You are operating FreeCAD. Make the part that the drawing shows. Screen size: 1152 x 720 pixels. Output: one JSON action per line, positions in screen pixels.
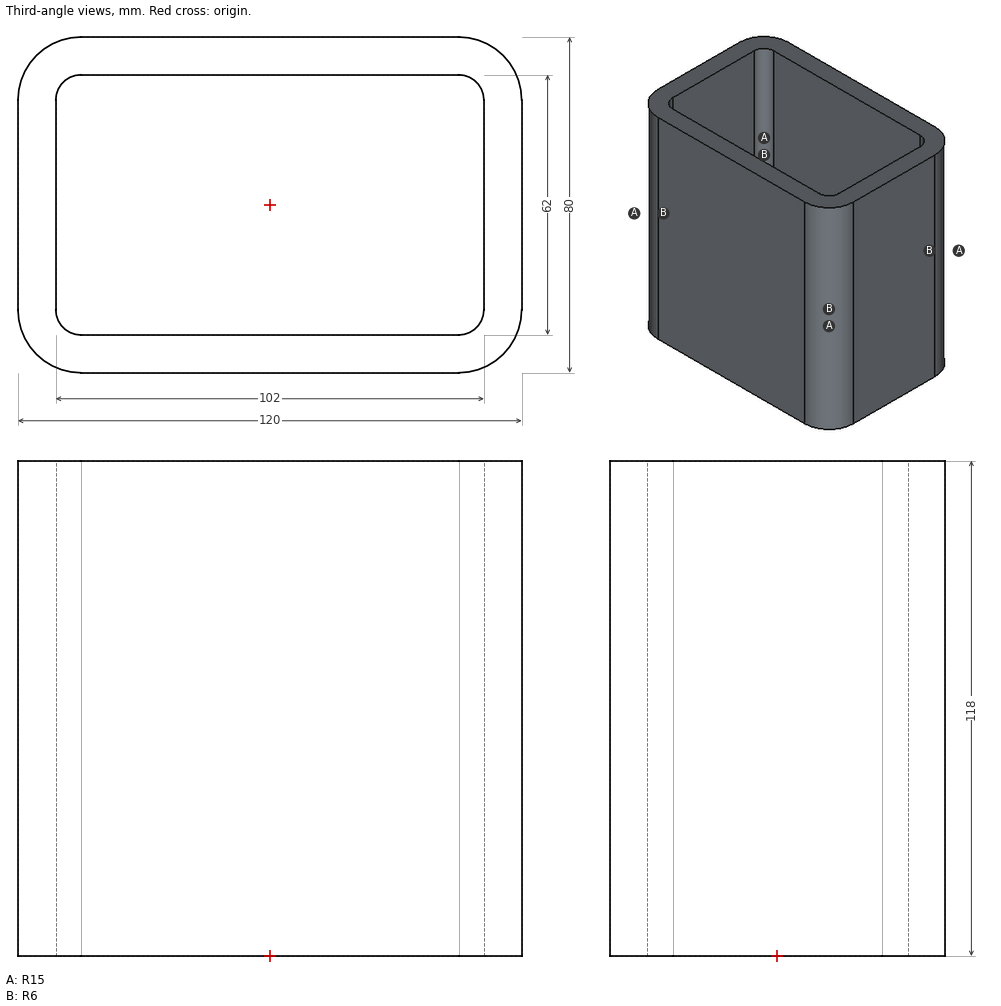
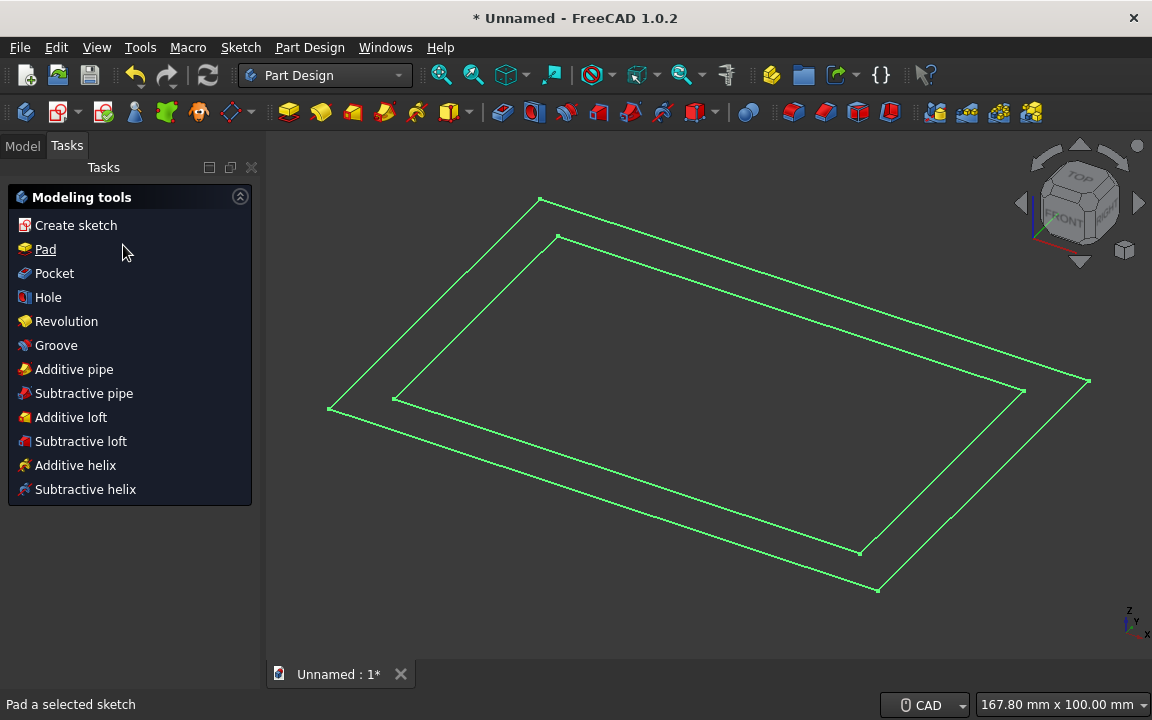
{"action": "left_click", "coordinate": [290, 112]}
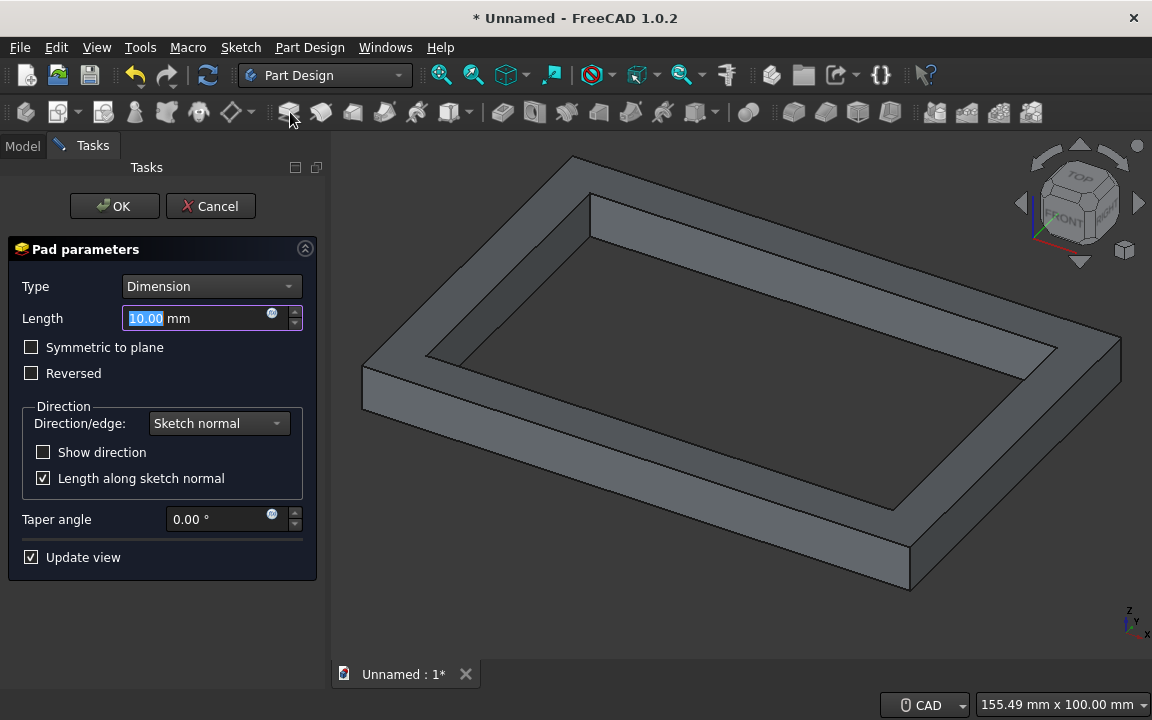
{"action": "type", "text": "118"}
{"action": "key", "text": "Tab"}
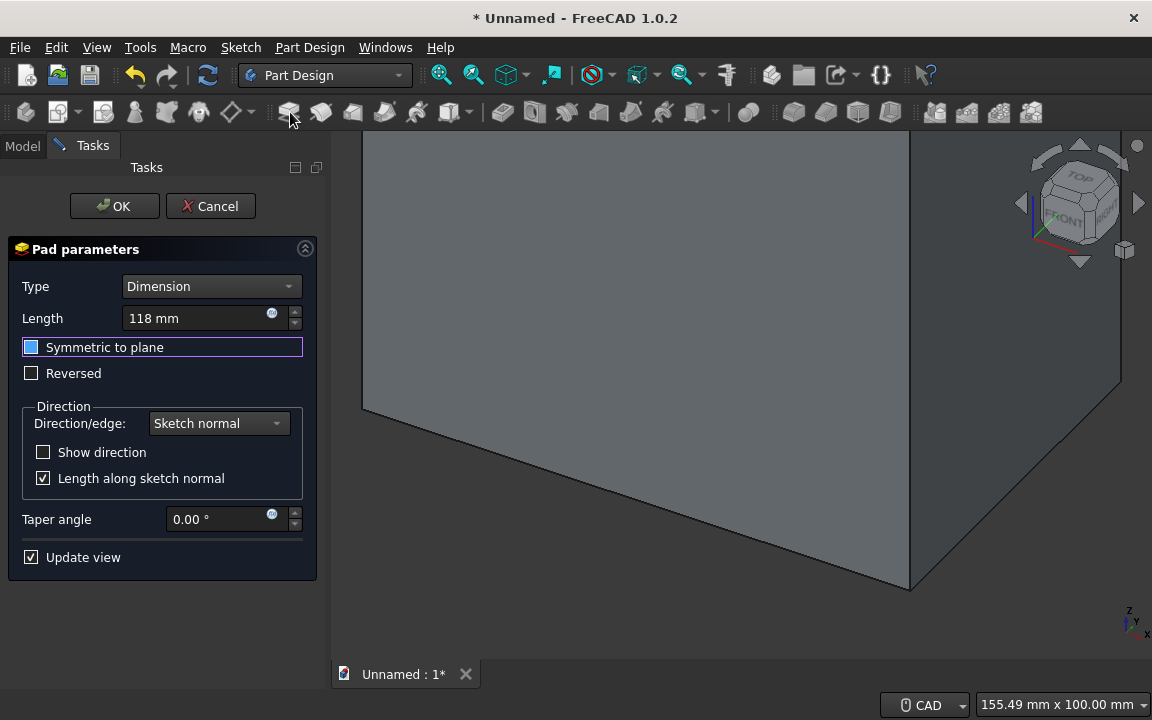
{"action": "left_click", "coordinate": [115, 206]}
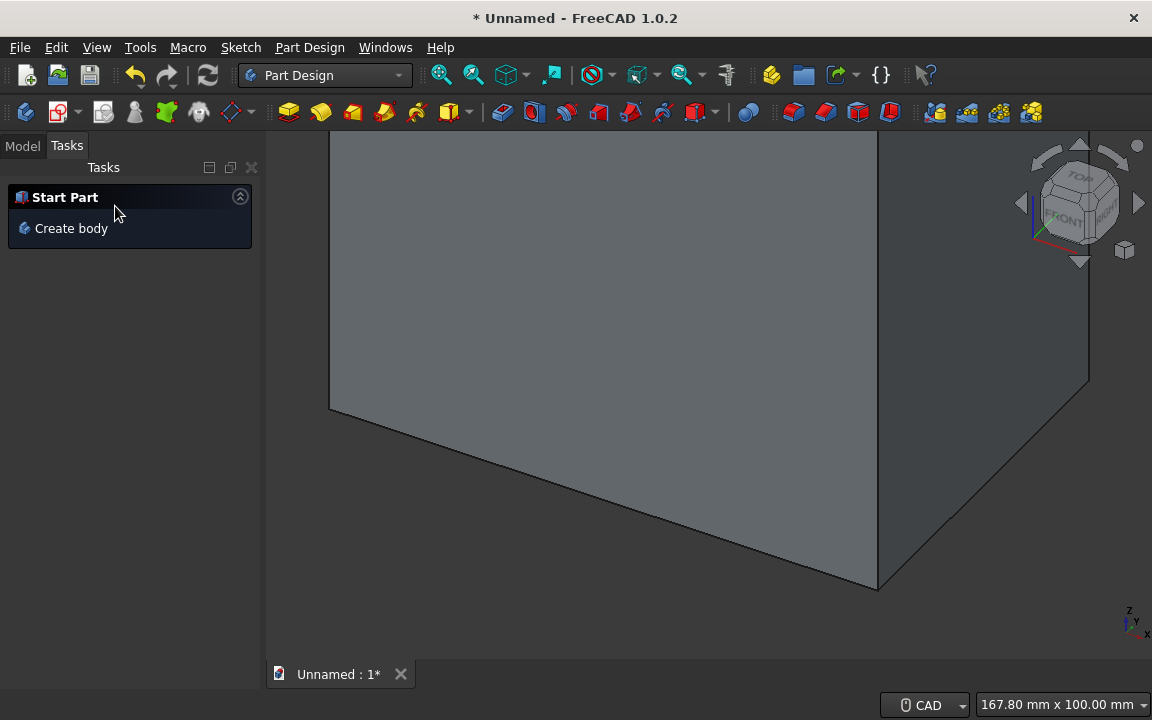
{"action": "left_click", "coordinate": [442, 76]}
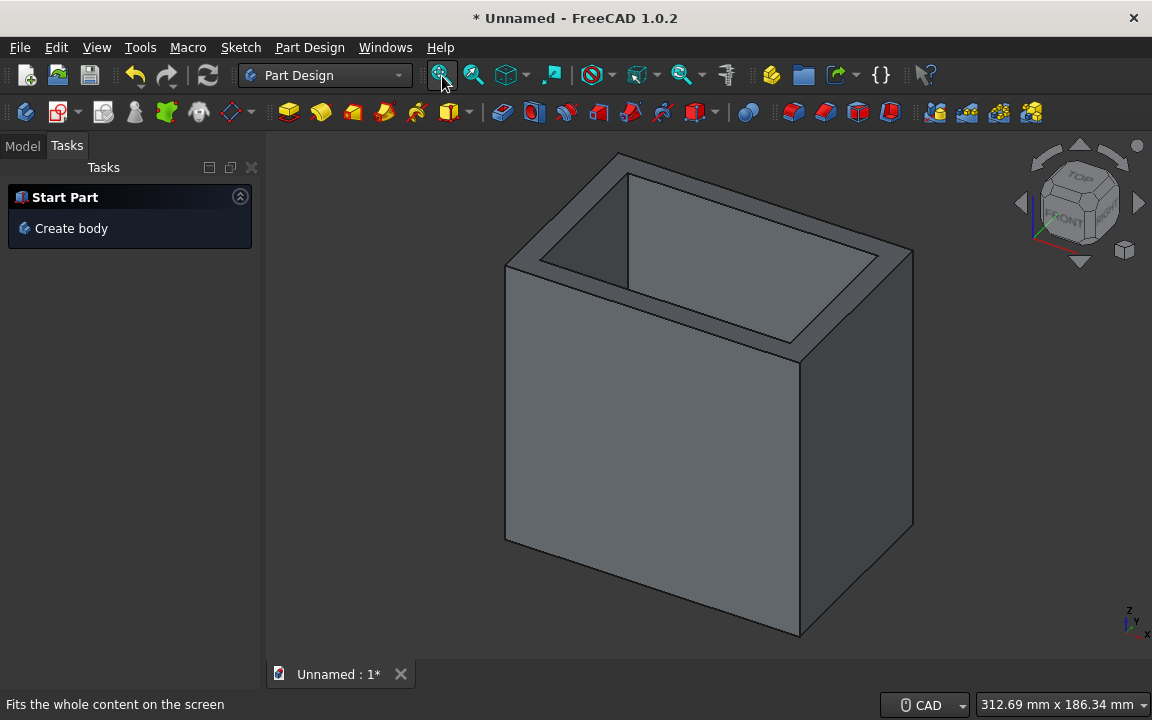
{"action": "left_click", "coordinate": [800, 499]}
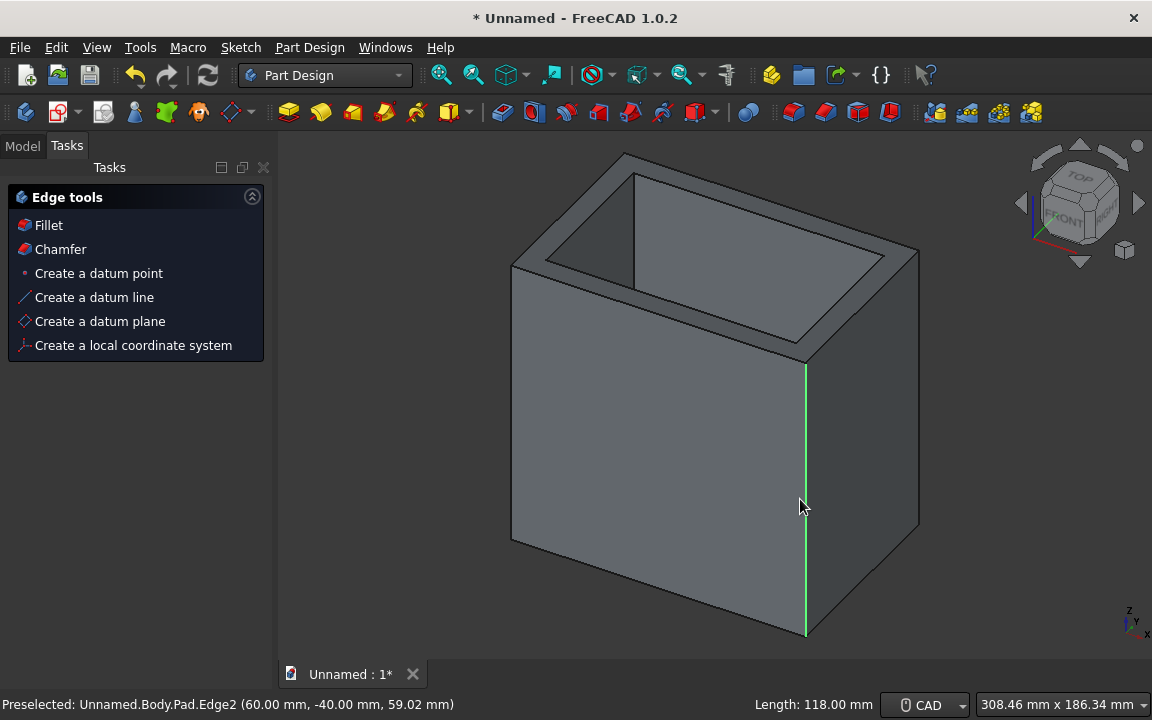
{"action": "key", "text": "0"}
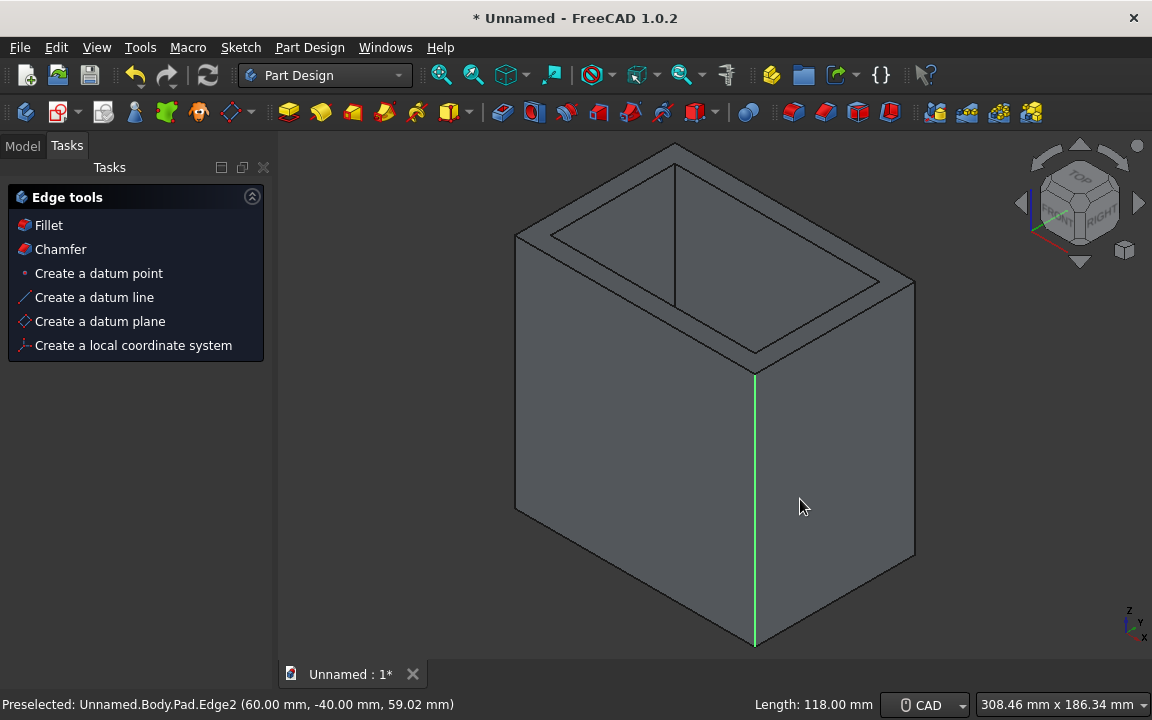
{"action": "key", "text": "2"}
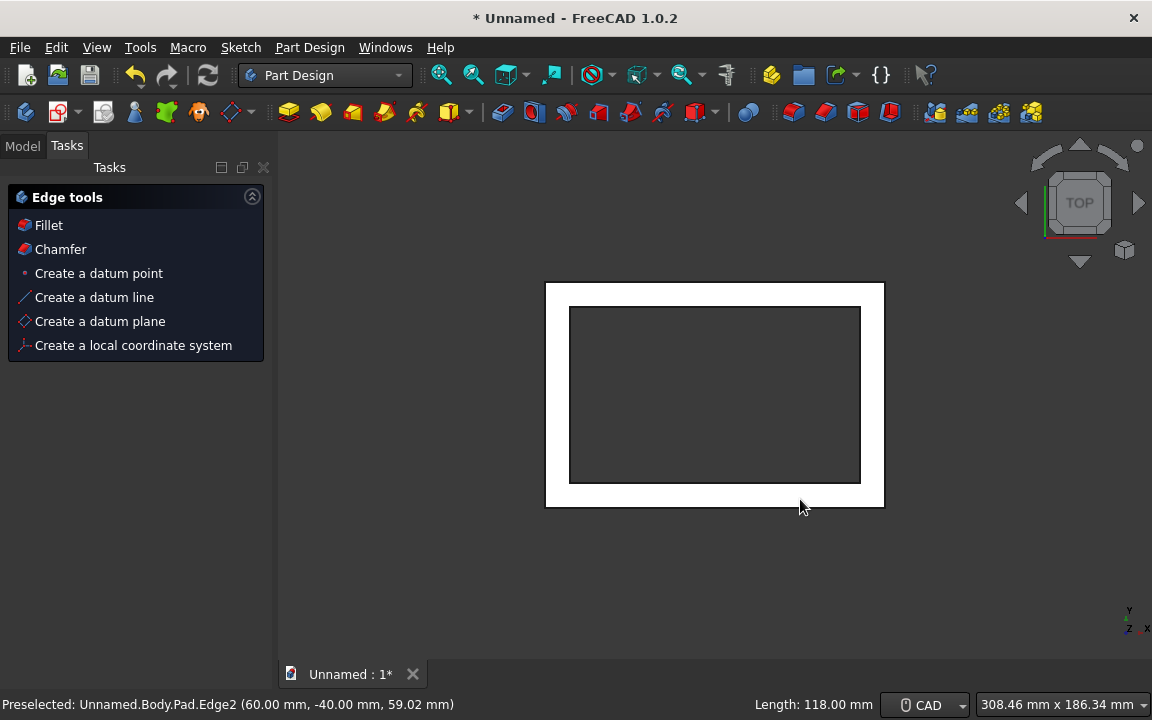
{"action": "left_click", "coordinate": [442, 76]}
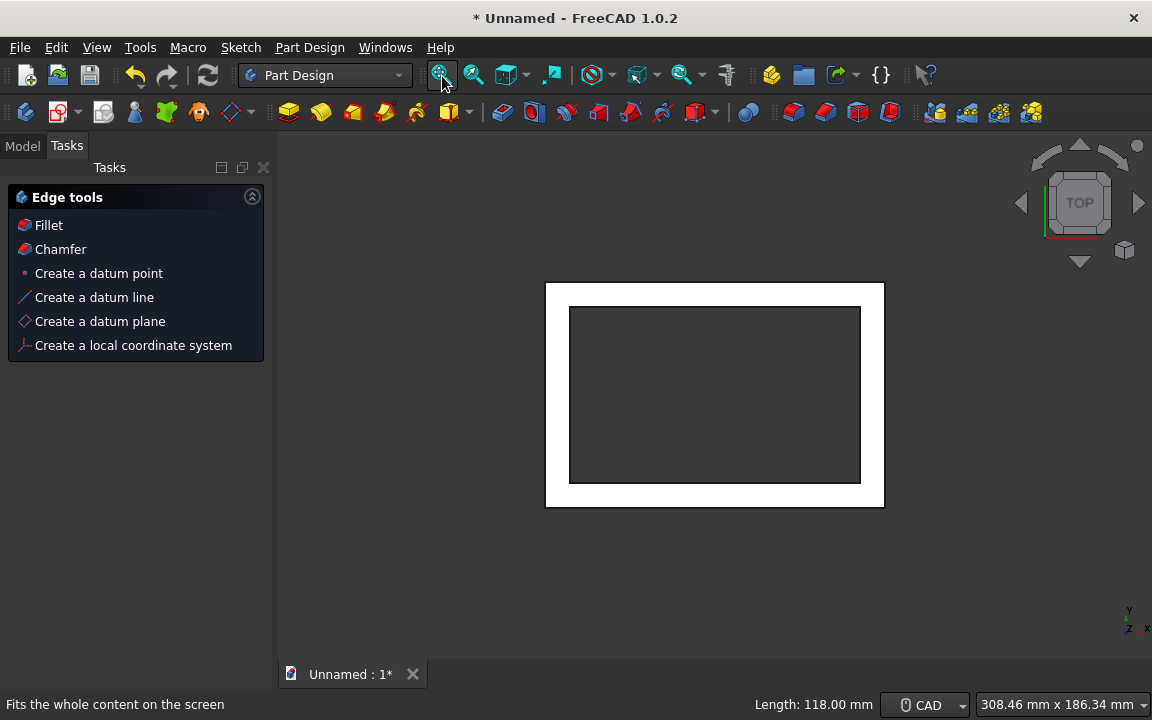
{"action": "key", "text": "1"}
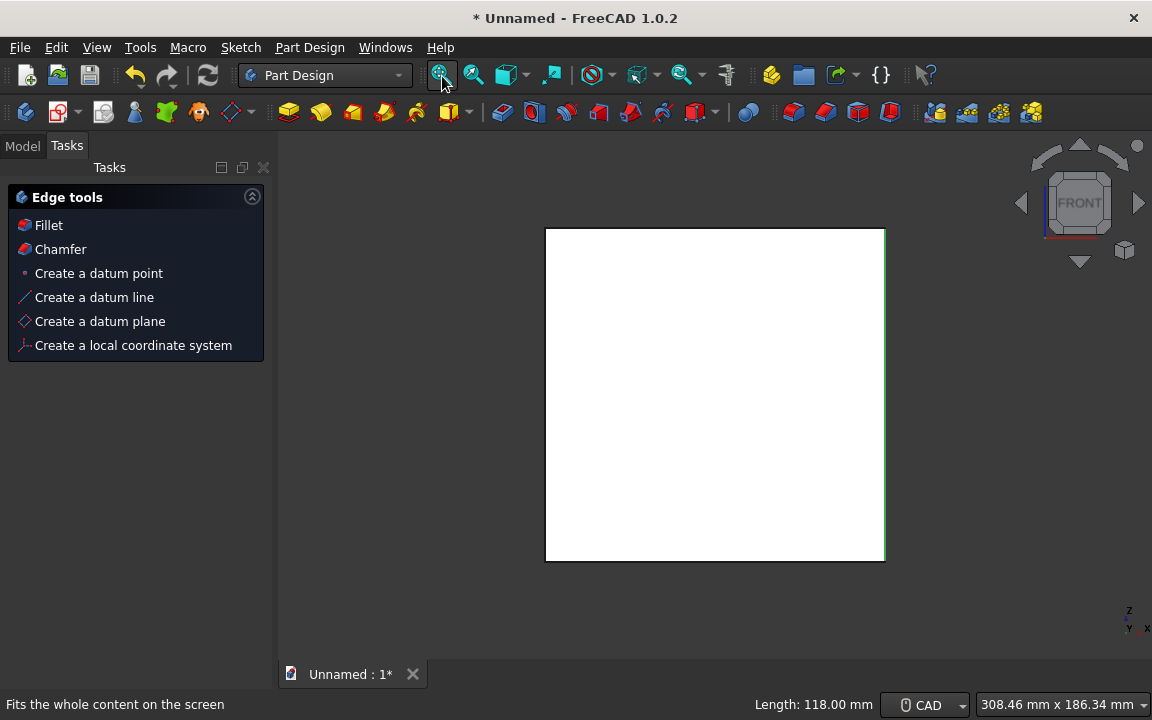
{"action": "left_click", "coordinate": [545, 394], "text": "ctrl"}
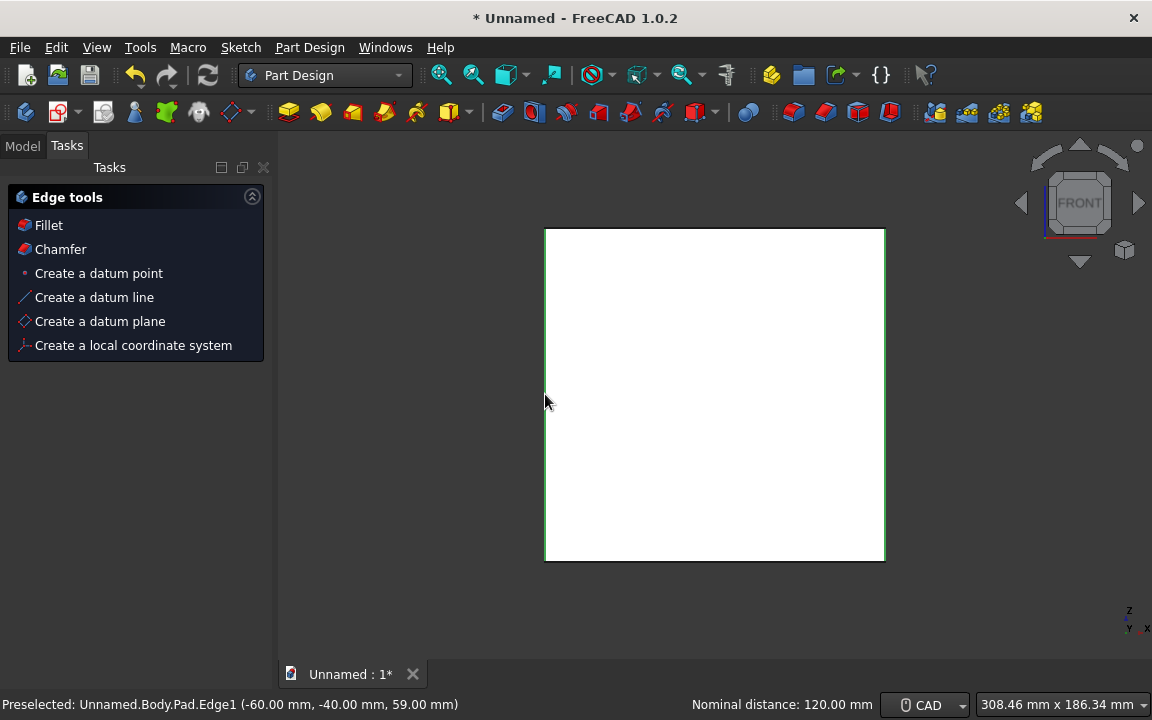
{"action": "key", "text": "3"}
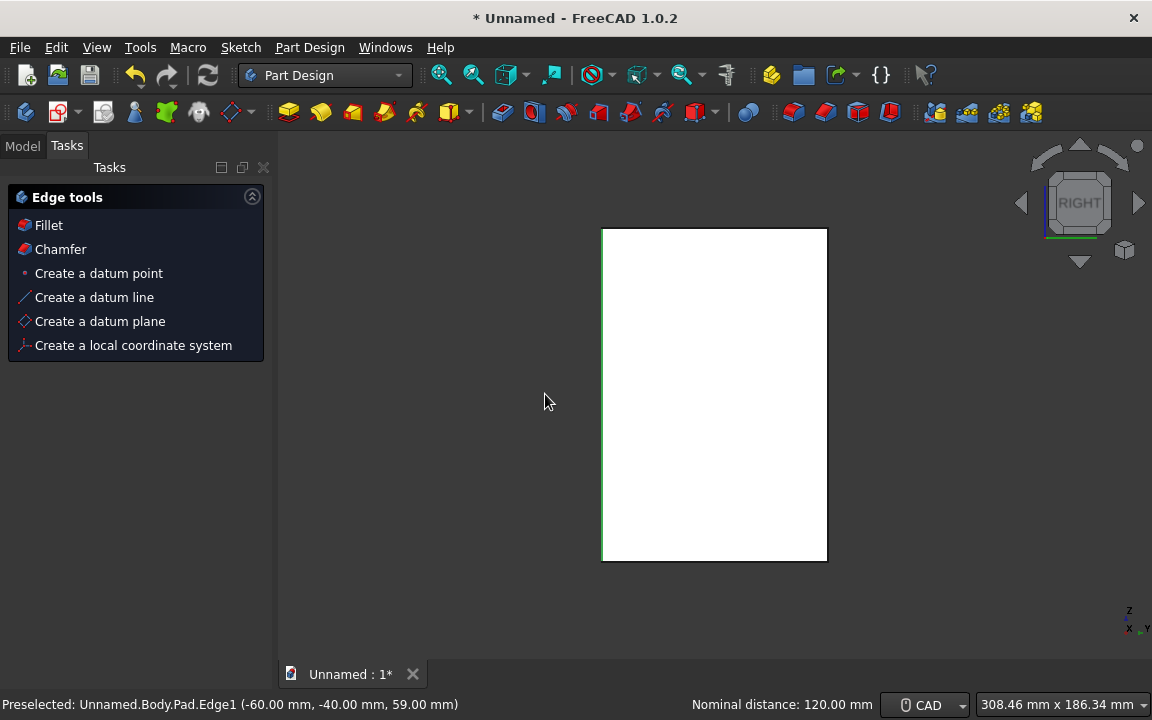
{"action": "left_click", "coordinate": [828, 394], "text": "ctrl"}